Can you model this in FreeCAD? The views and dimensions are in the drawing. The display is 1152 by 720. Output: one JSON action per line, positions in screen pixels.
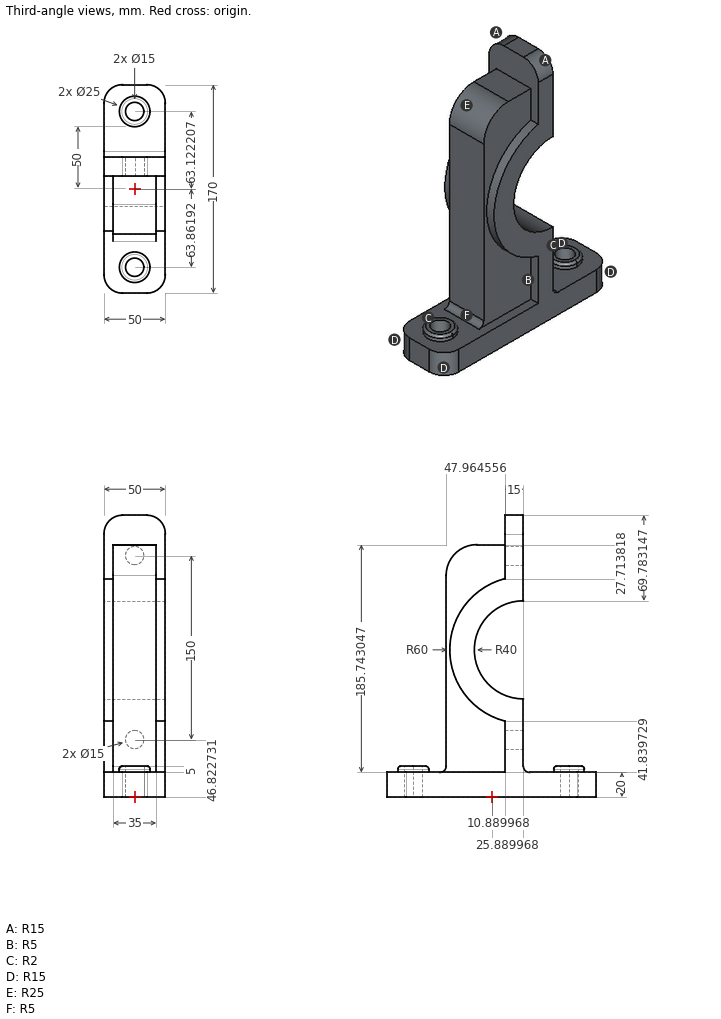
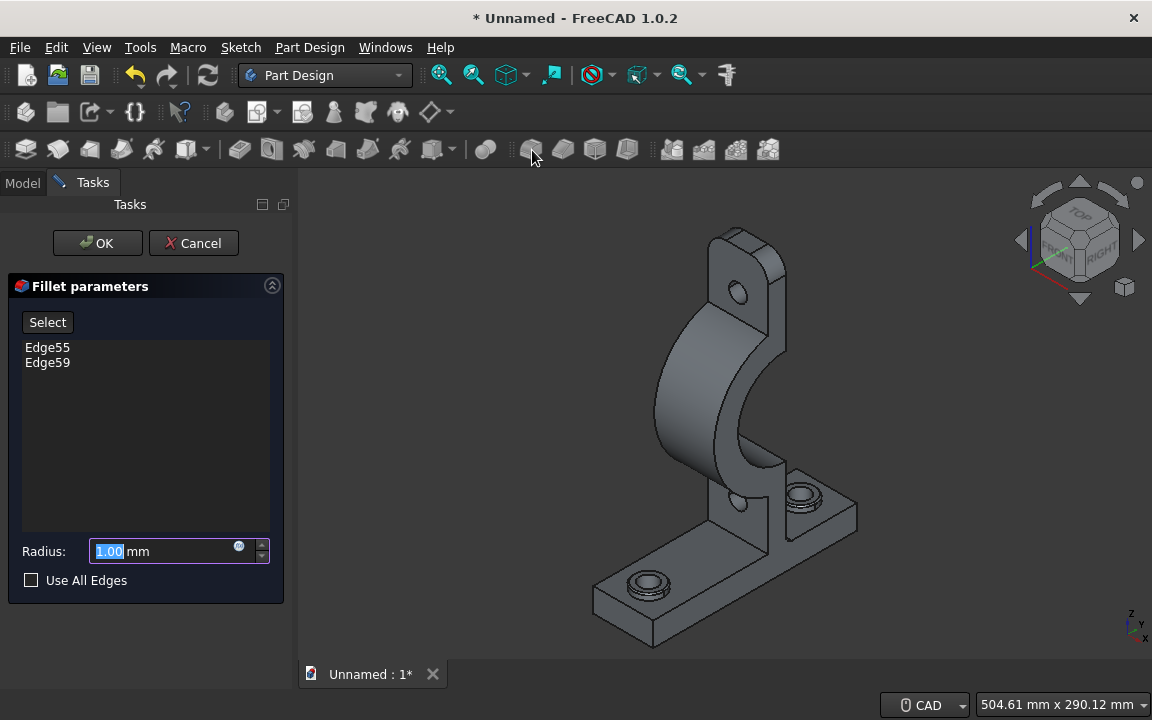
{"action": "type", "text": "2"}
{"action": "key", "text": "Tab"}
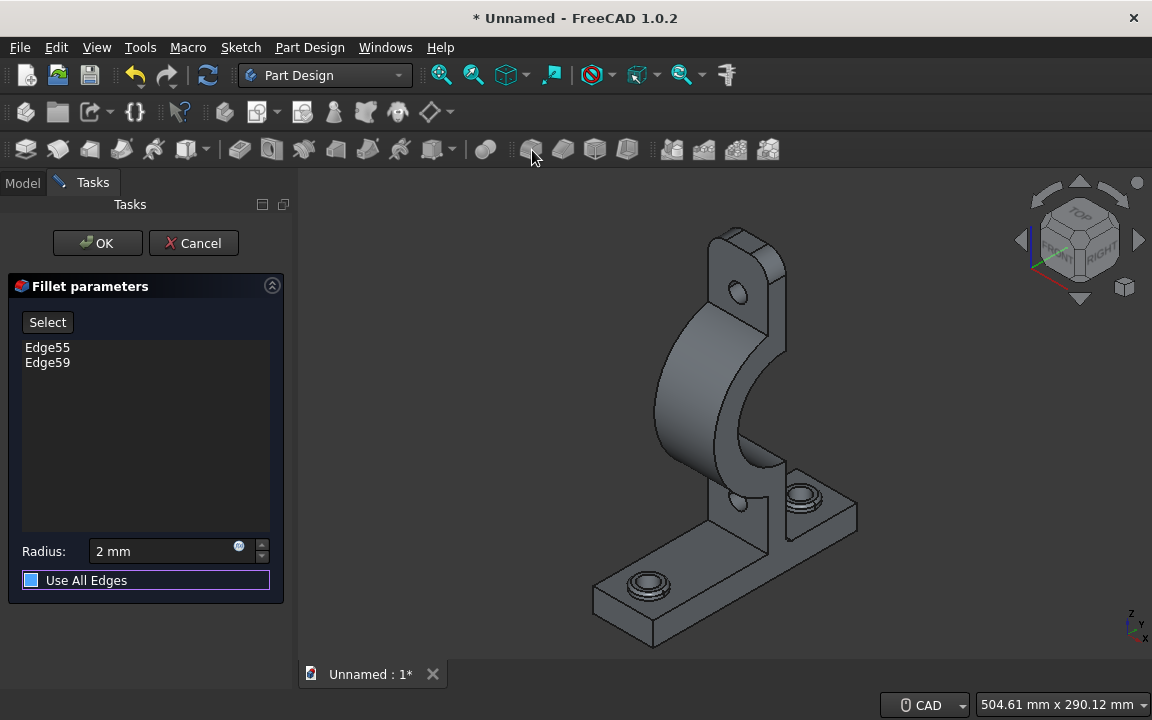
{"action": "left_click", "coordinate": [98, 243]}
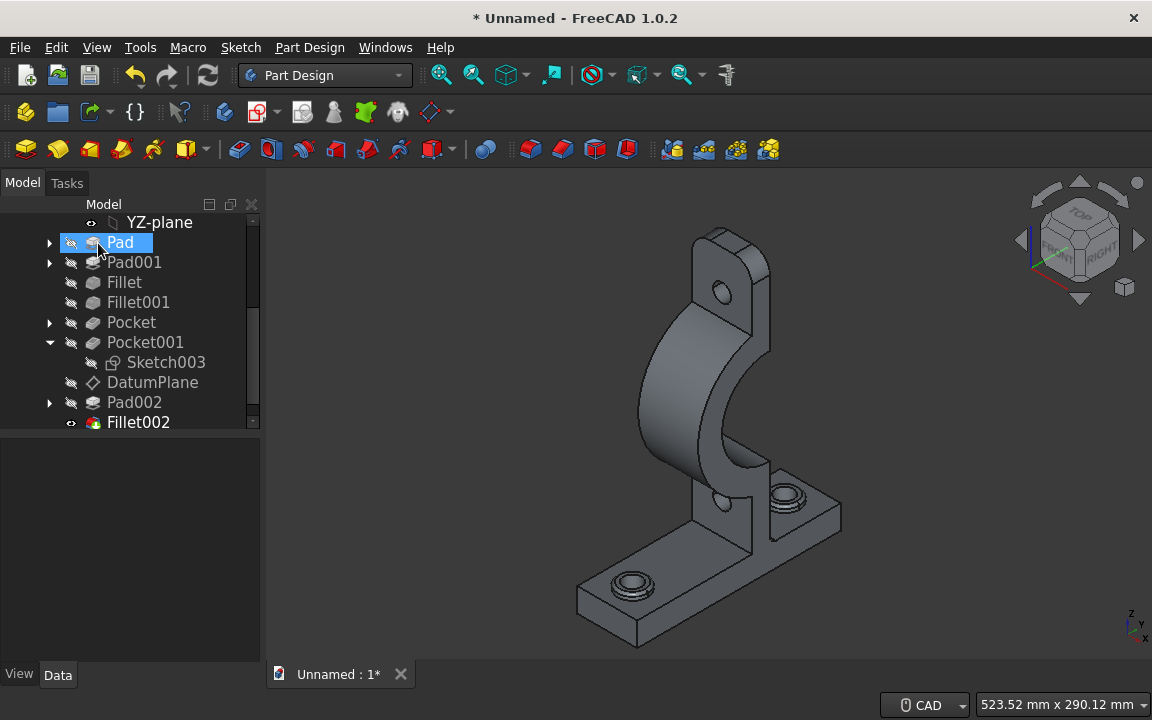
{"action": "left_click", "coordinate": [637, 628]}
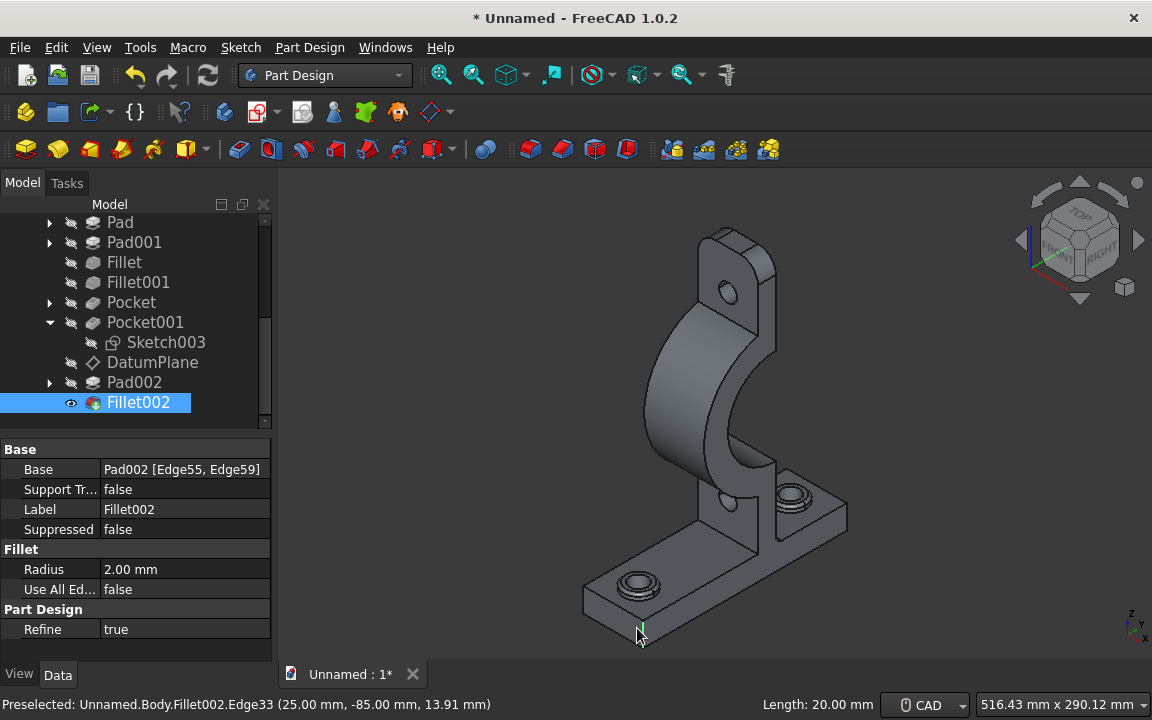
{"action": "key", "text": "2"}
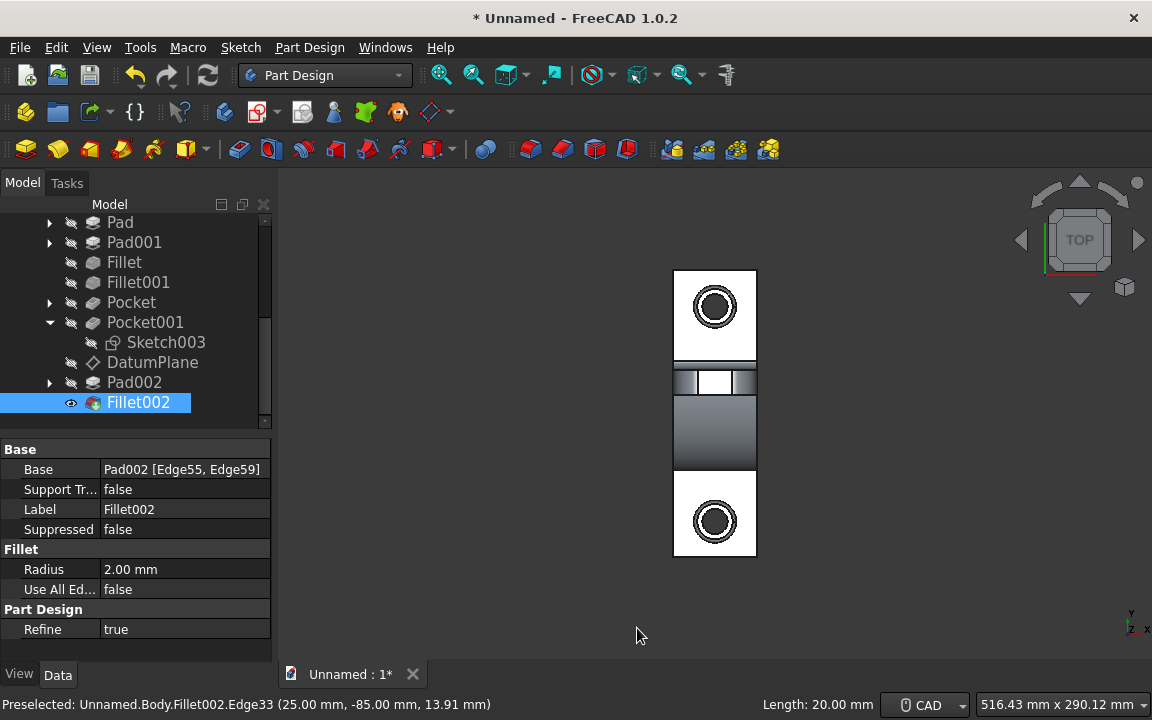
{"action": "key", "text": "0"}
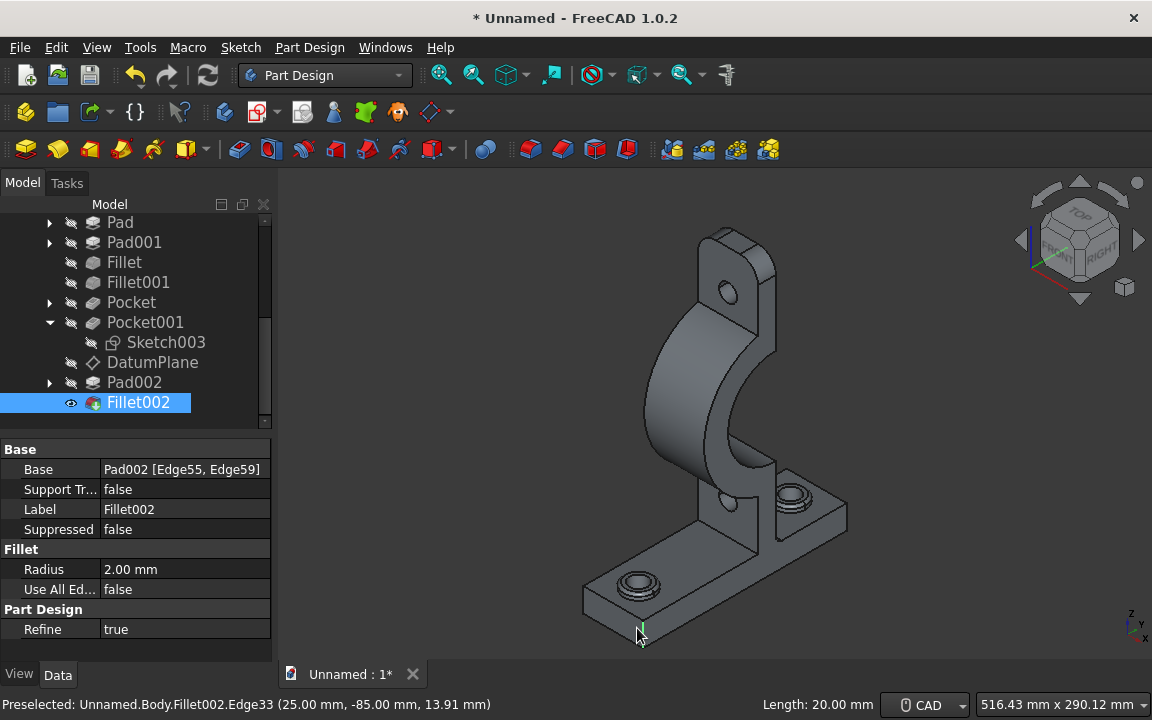
{"action": "key", "text": "1"}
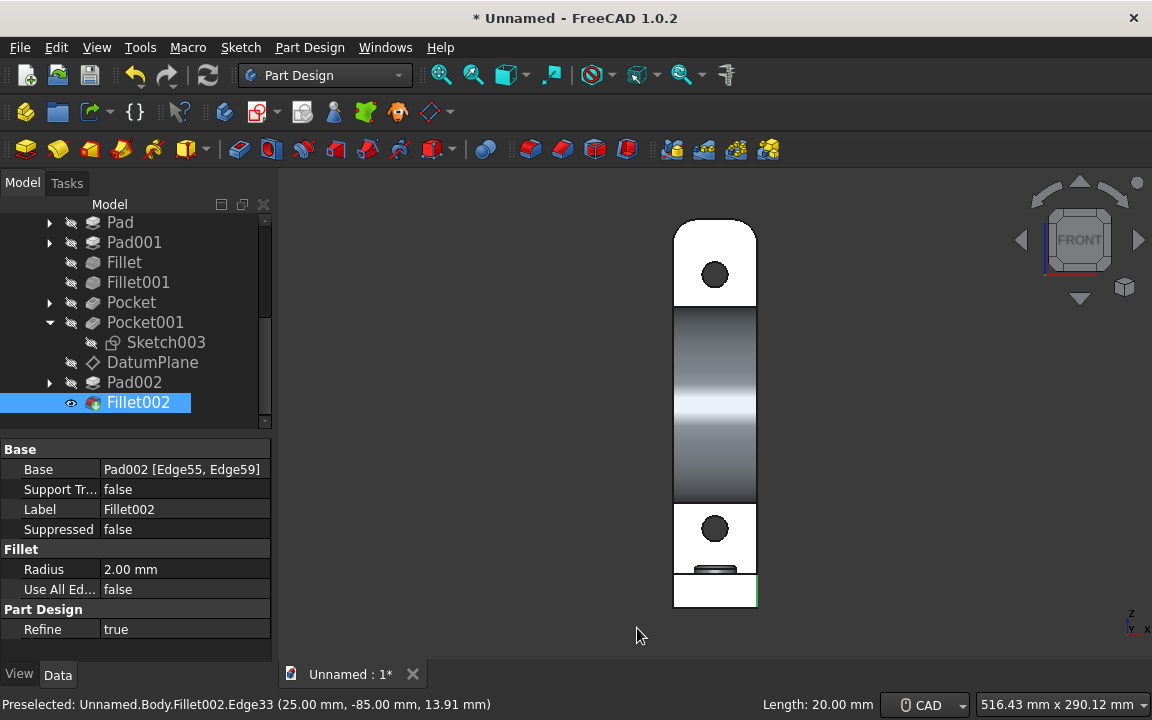
{"action": "left_click", "coordinate": [673, 590], "text": "ctrl"}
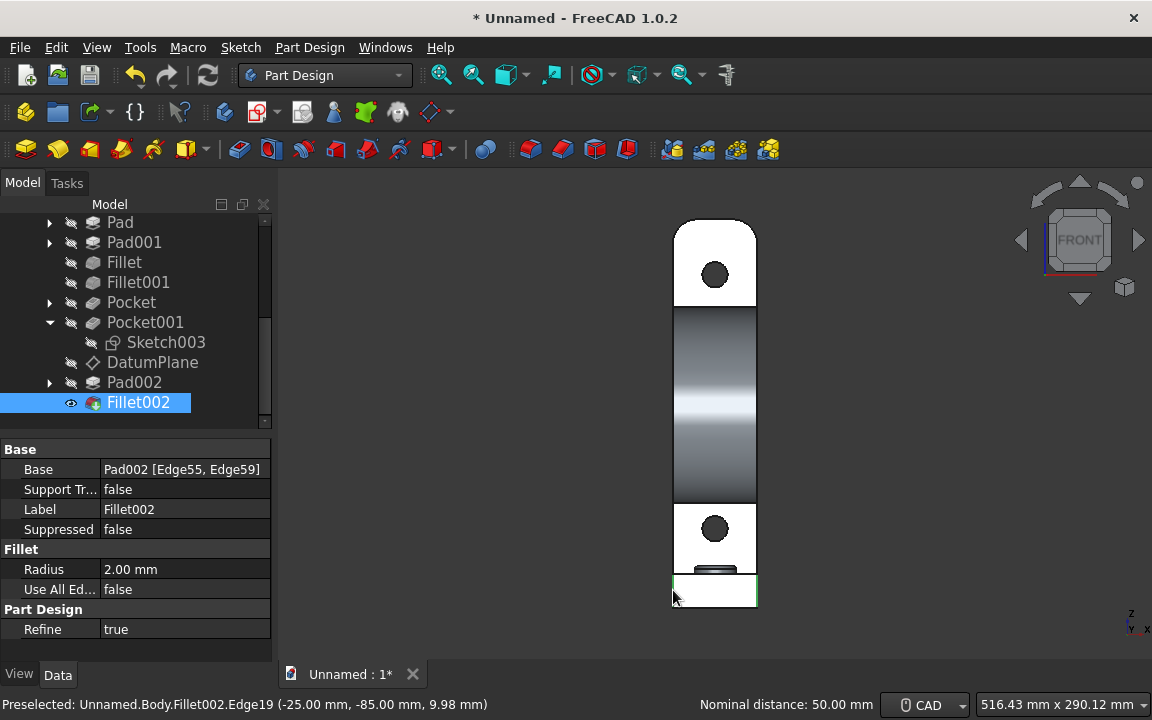
{"action": "key", "text": "3"}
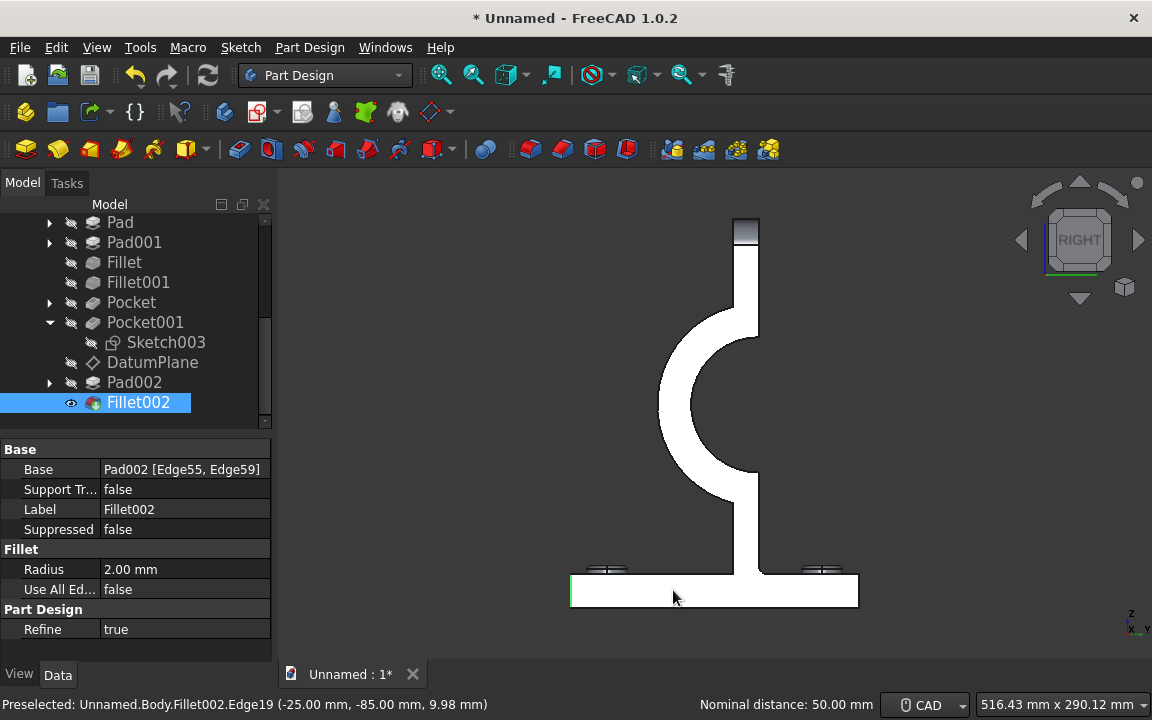
{"action": "left_click", "coordinate": [859, 590], "text": "ctrl"}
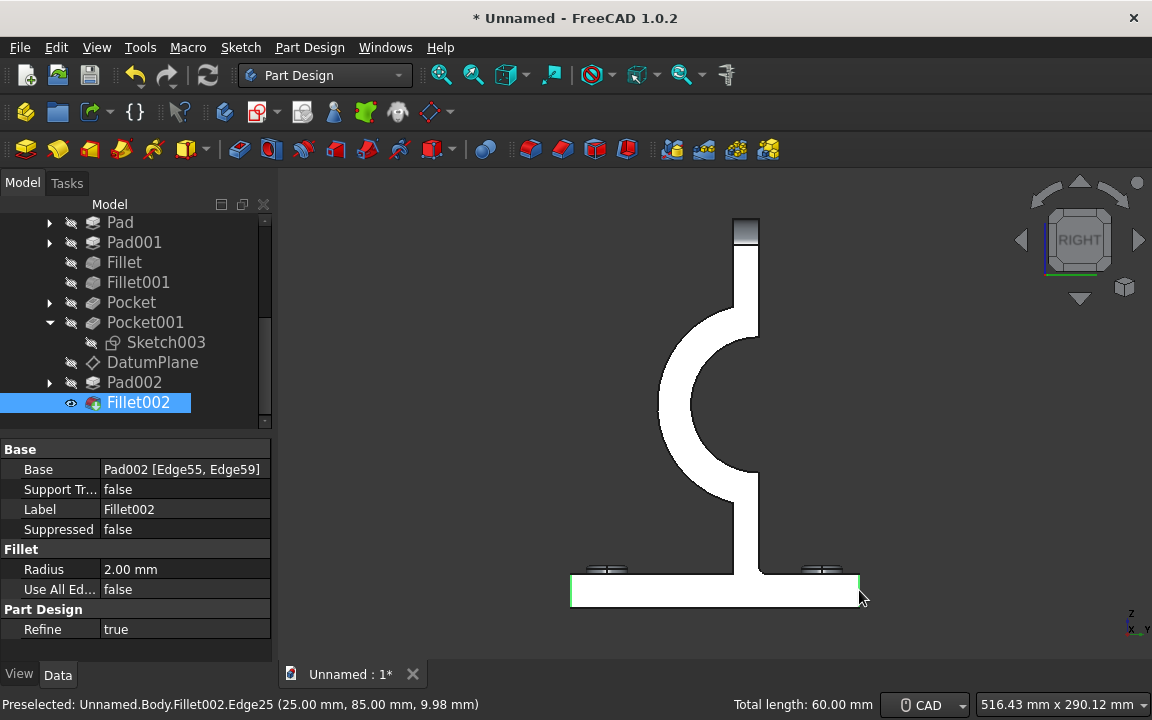
{"action": "key", "text": "5"}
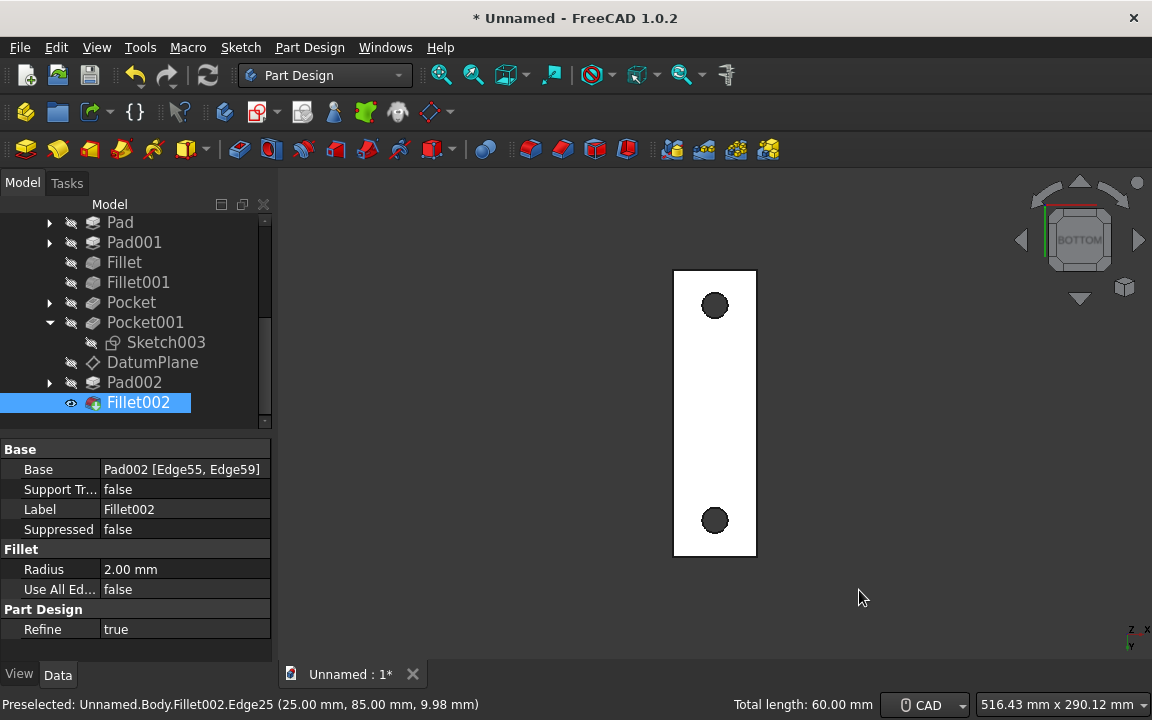
{"action": "key", "text": "4"}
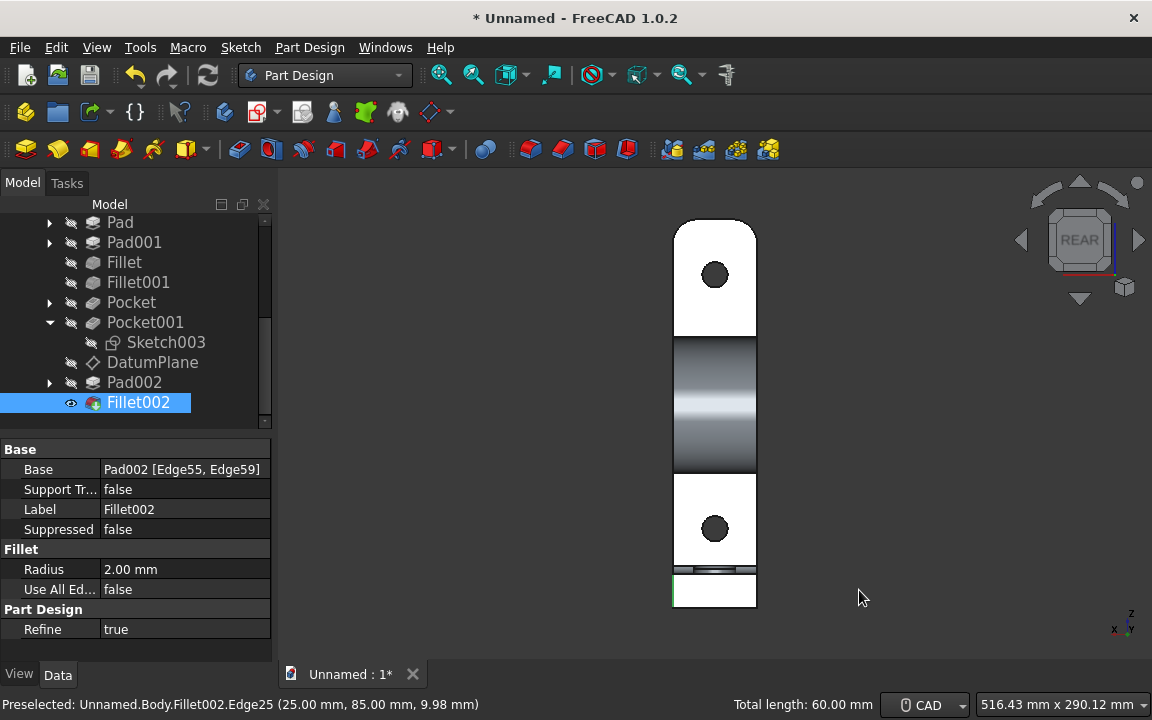
{"action": "left_click", "coordinate": [757, 590], "text": "ctrl"}